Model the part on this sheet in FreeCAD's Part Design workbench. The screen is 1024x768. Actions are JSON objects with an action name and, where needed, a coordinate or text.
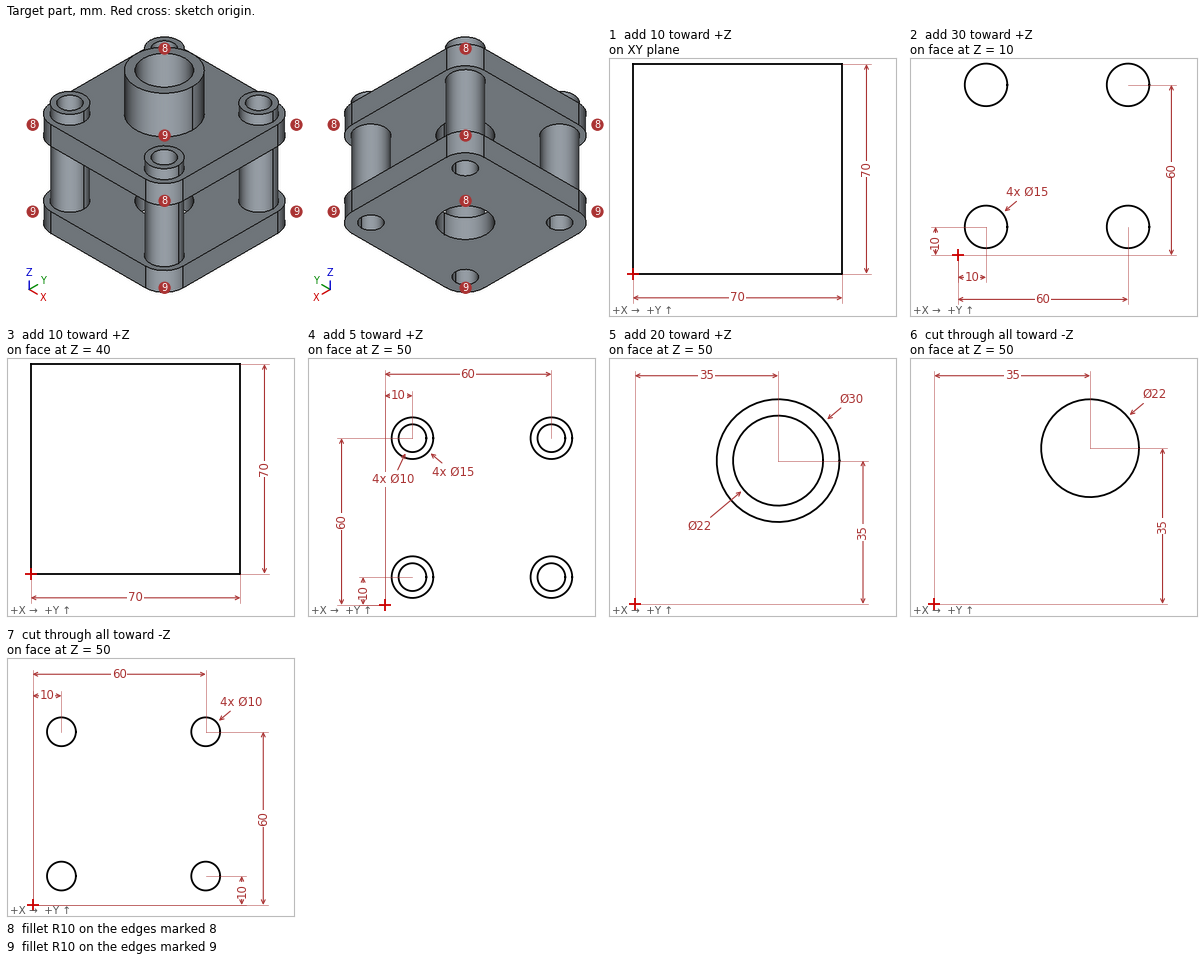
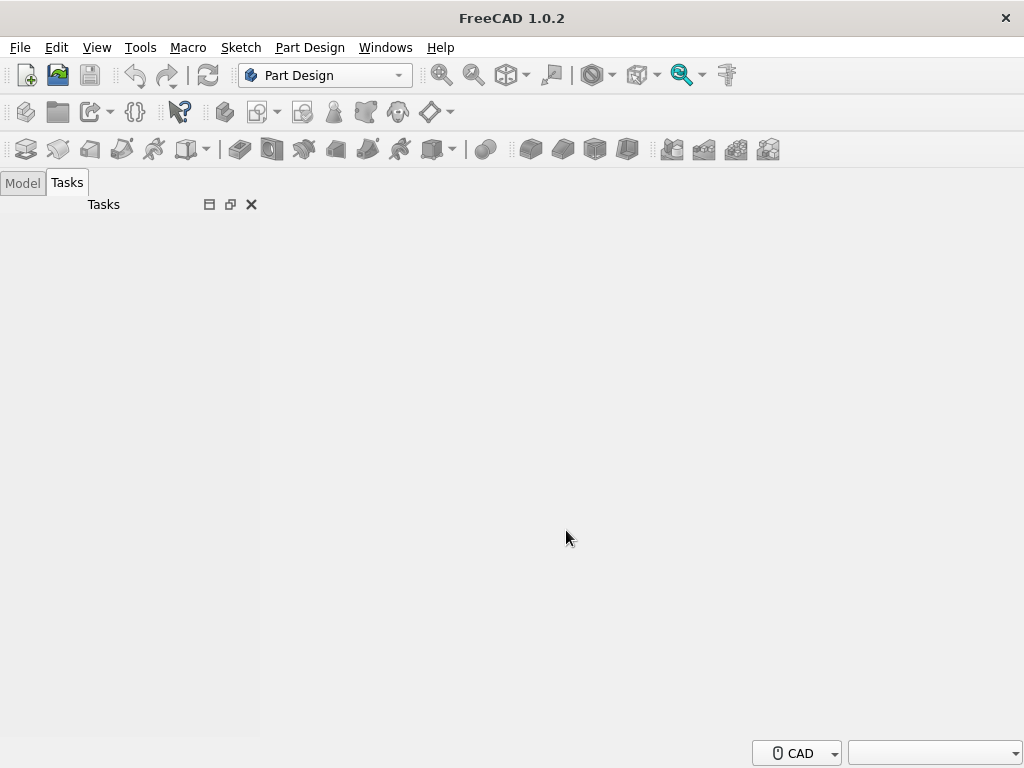
{"action": "key", "text": "ctrl+n"}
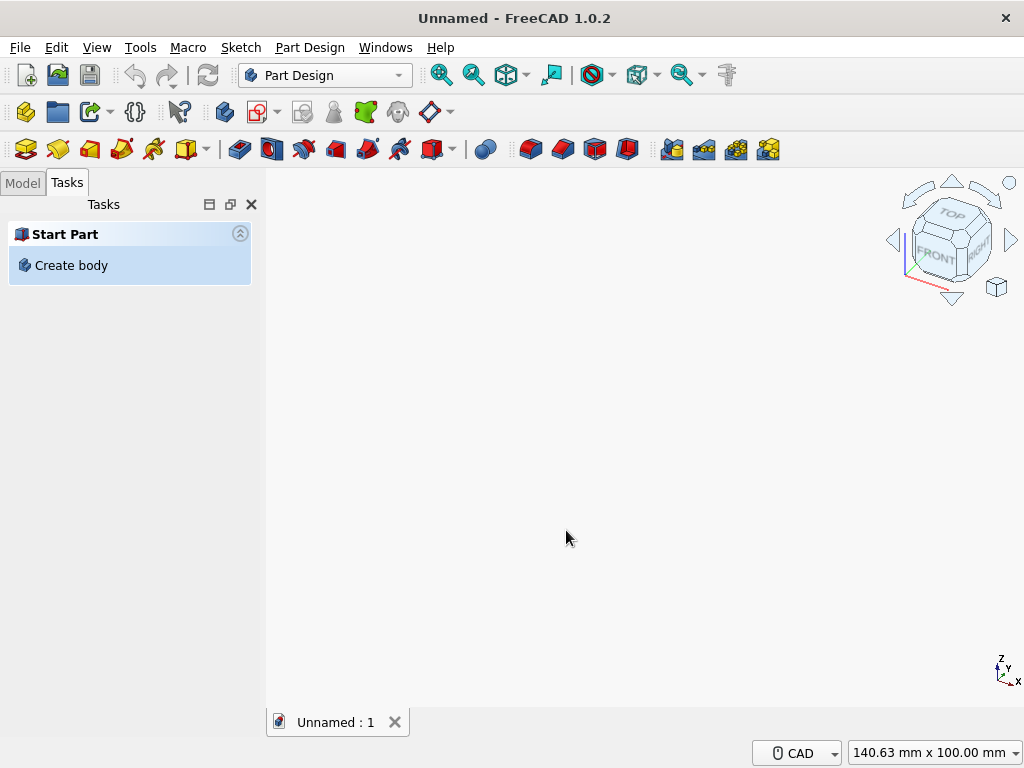
{"action": "left_click", "coordinate": [258, 112]}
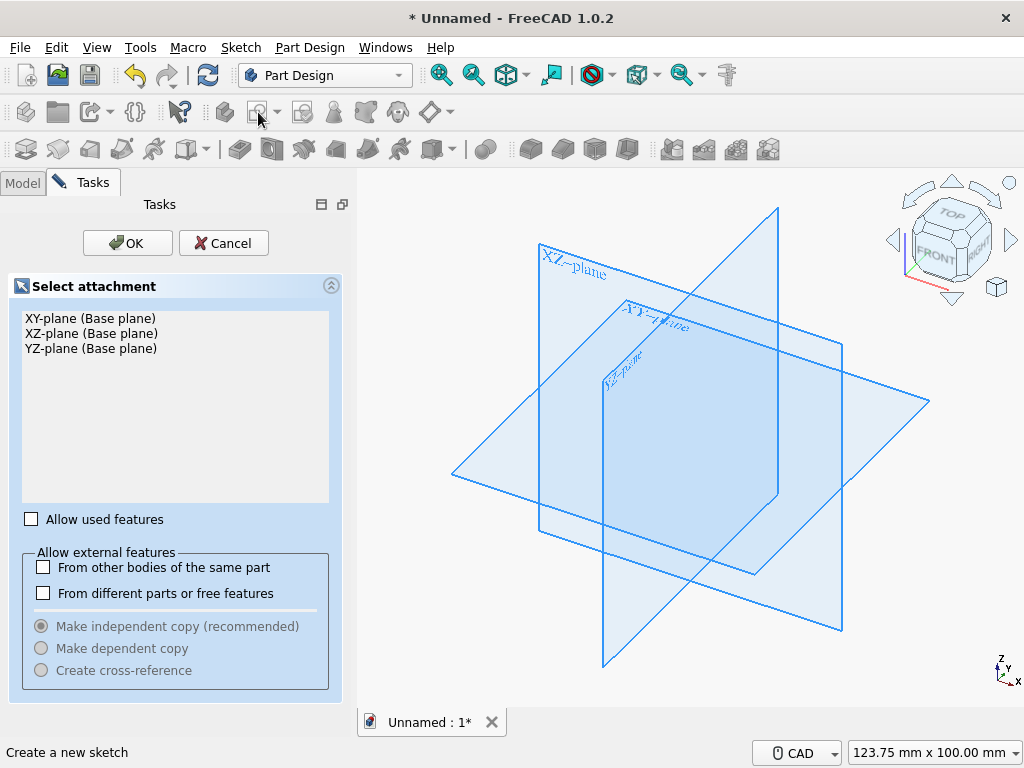
{"action": "left_click", "coordinate": [82, 318]}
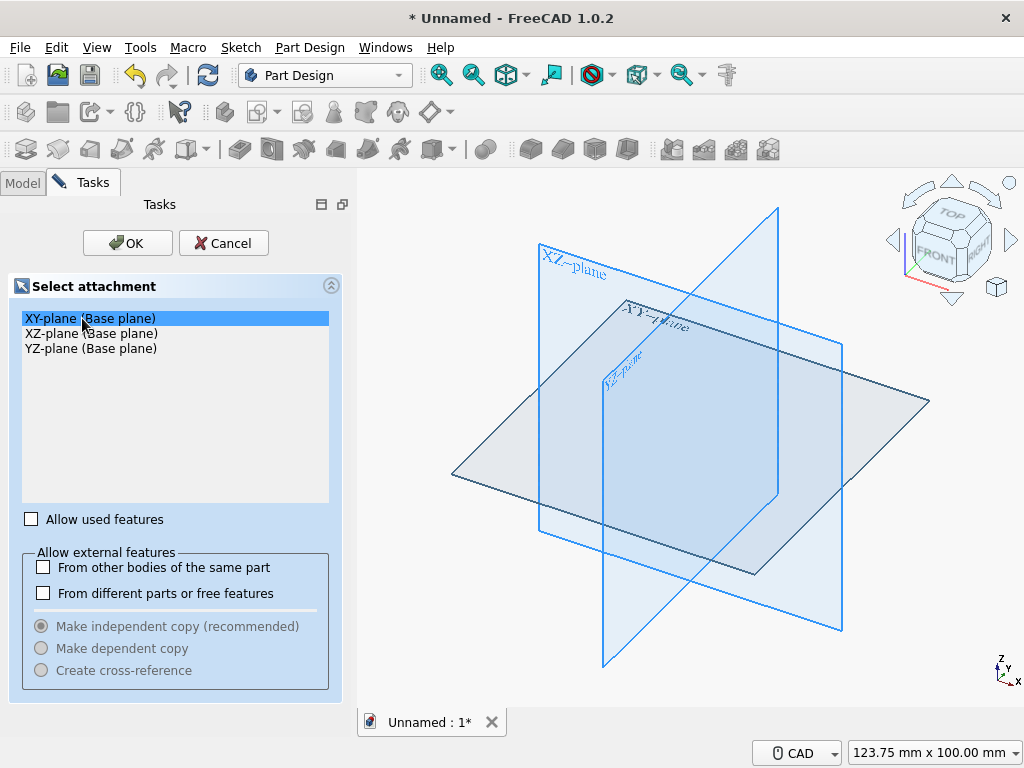
{"action": "left_click", "coordinate": [128, 243]}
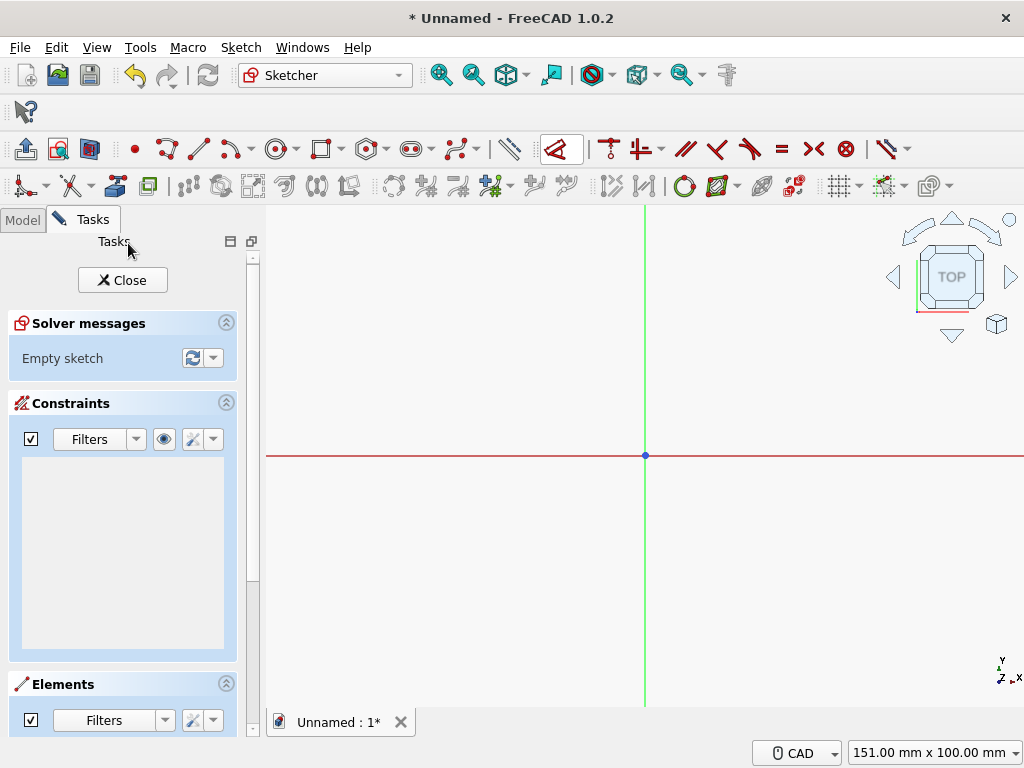
{"action": "scroll", "coordinate": [294, 679], "scroll_direction": "down", "scroll_amount": 2}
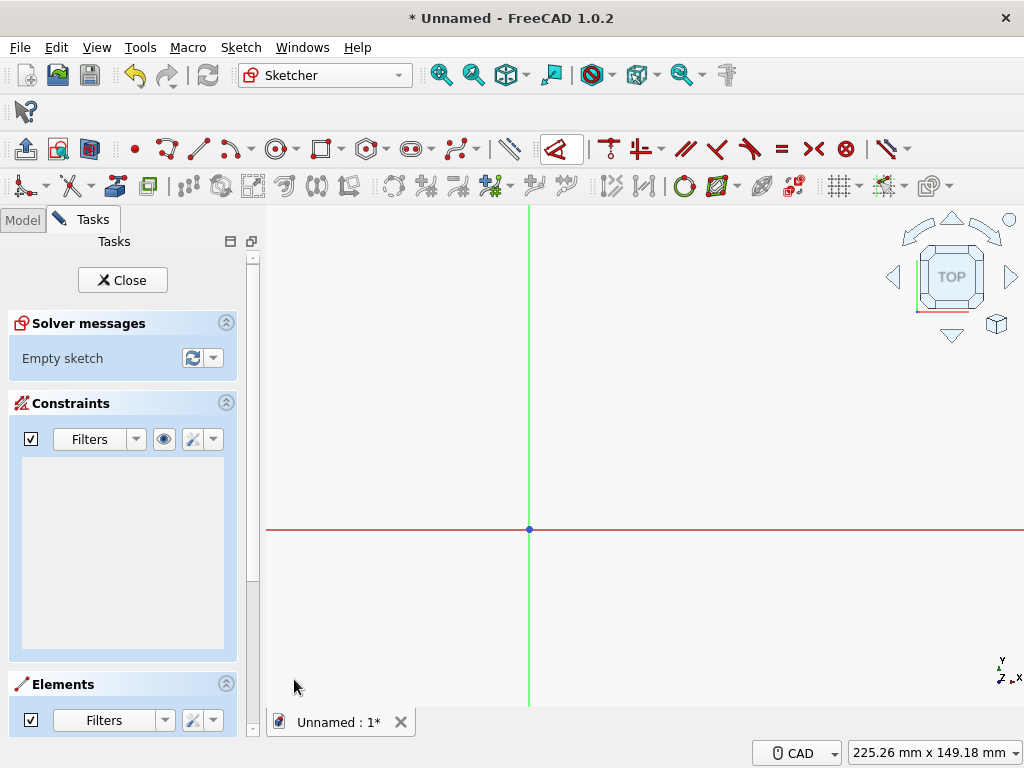
{"action": "key", "text": "g r"}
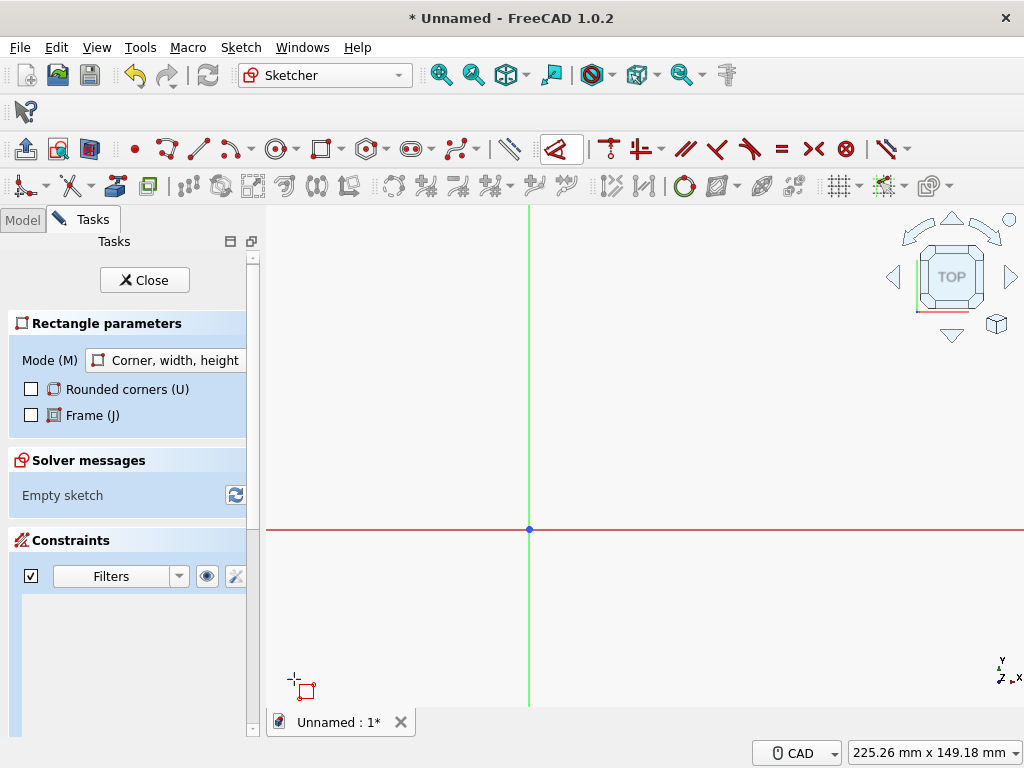
{"action": "left_click", "coordinate": [529, 530]}
{"action": "left_click", "coordinate": [765, 294]}
{"action": "key", "text": "Escape"}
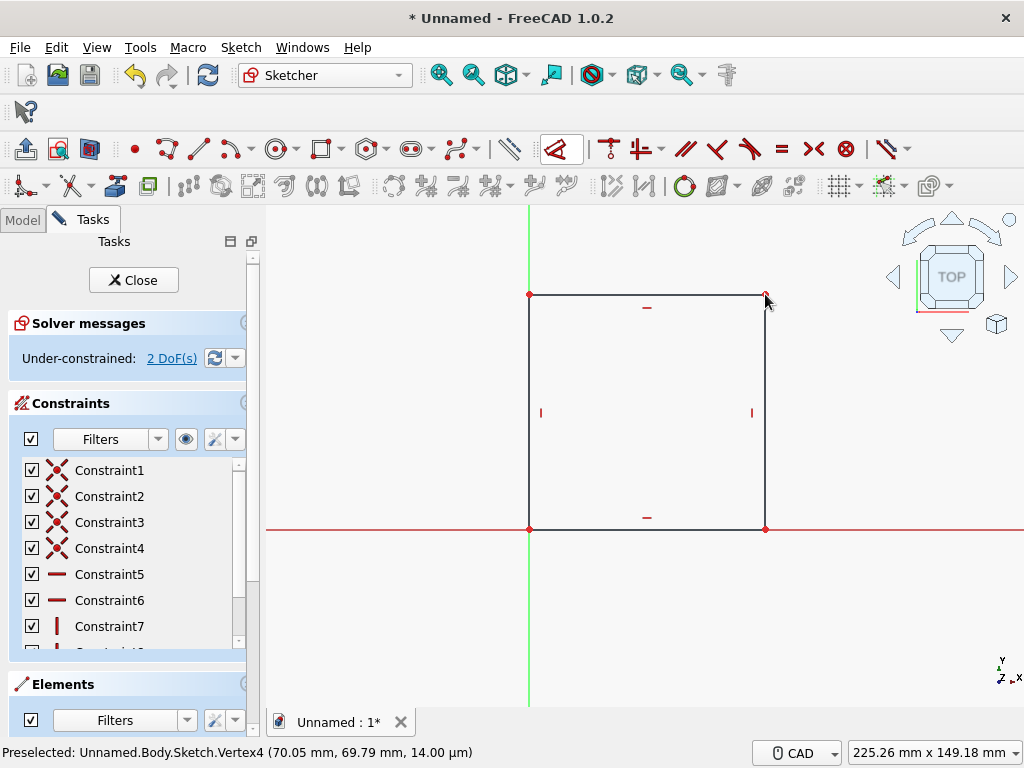
{"action": "left_click", "coordinate": [556, 150]}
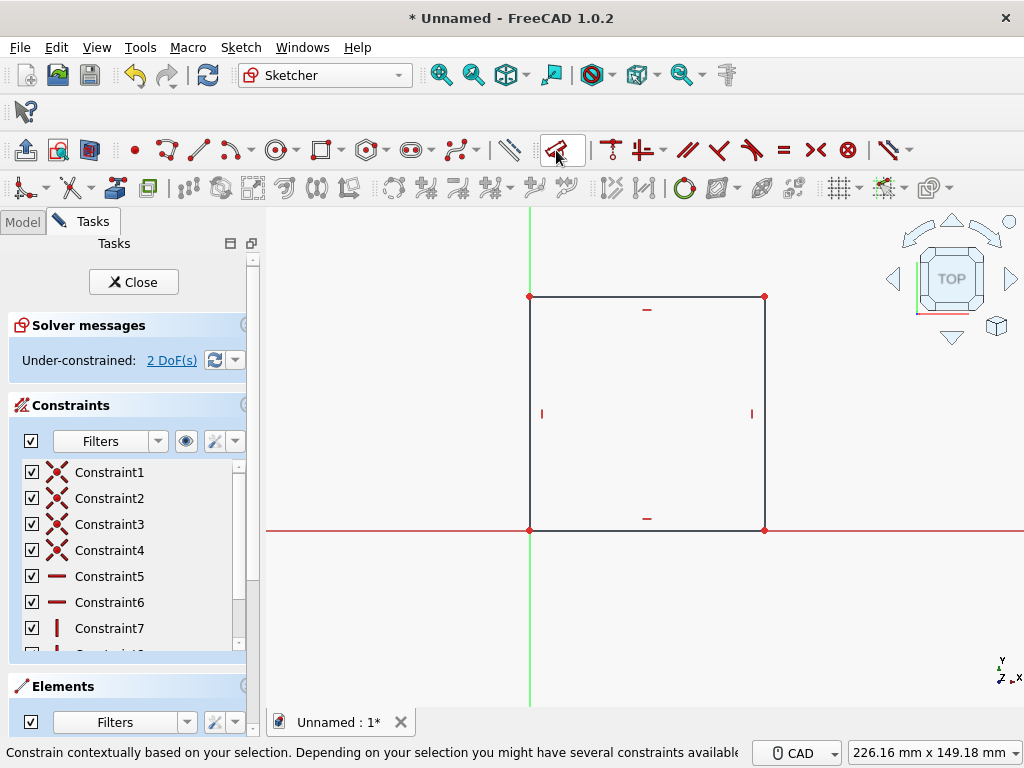
{"action": "left_click", "coordinate": [600, 531]}
{"action": "left_click", "coordinate": [647, 565]}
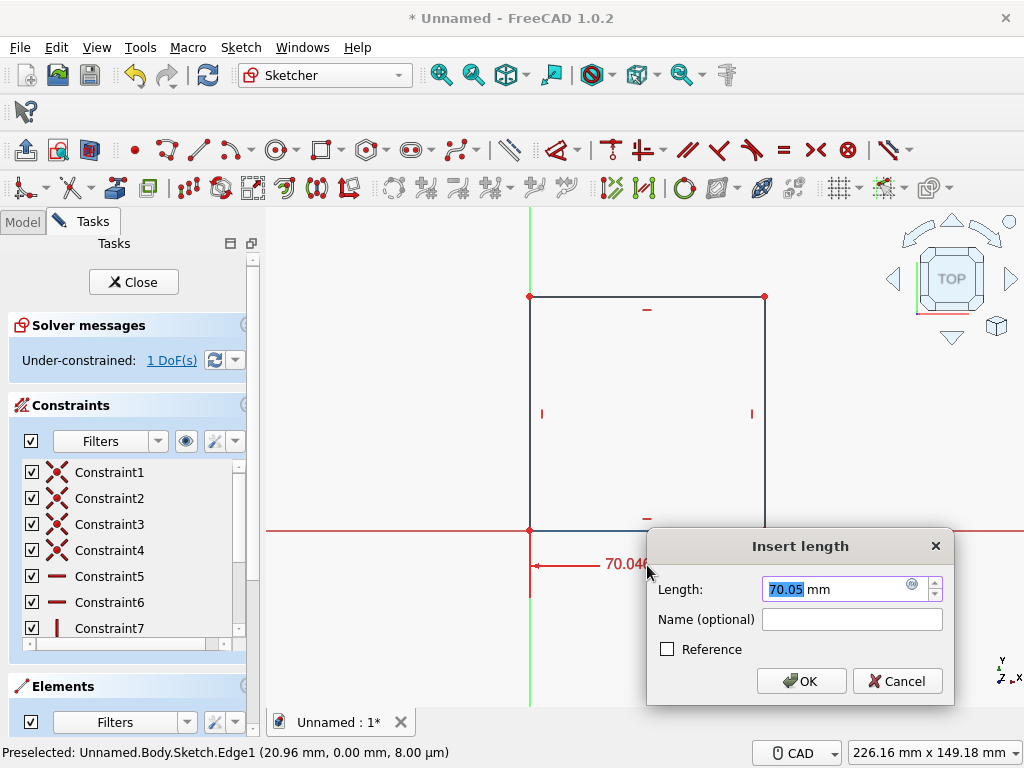
{"action": "type", "text": "70"}
{"action": "key", "text": "Return"}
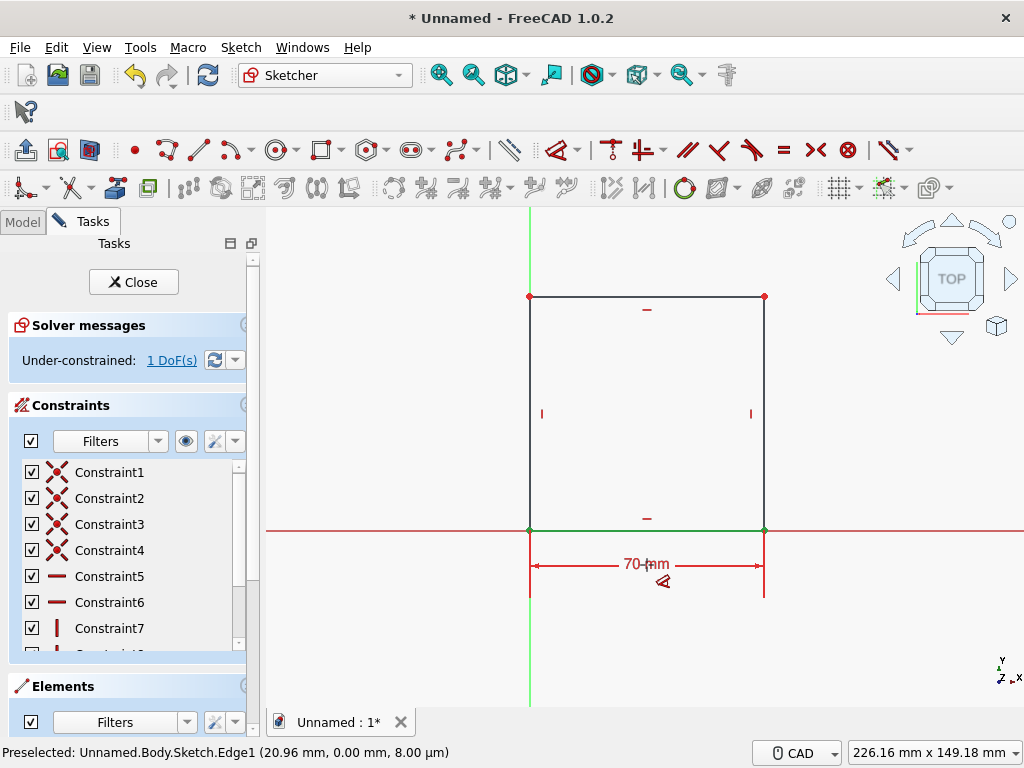
{"action": "left_click", "coordinate": [764, 460]}
{"action": "left_click", "coordinate": [798, 414]}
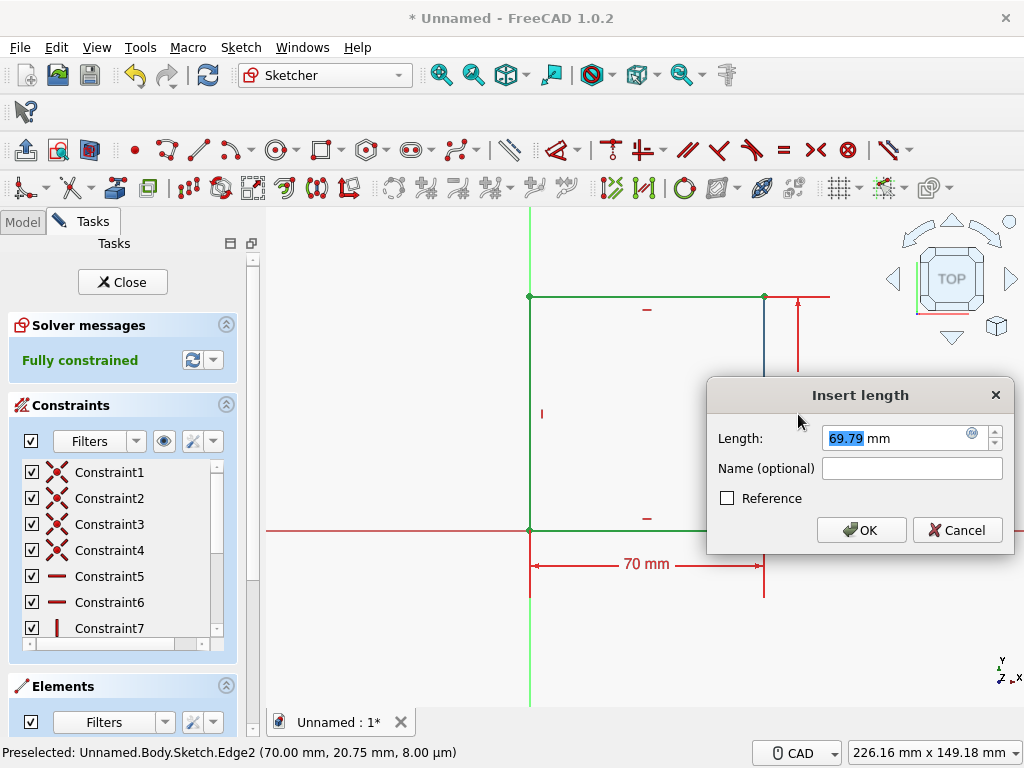
{"action": "type", "text": "70"}
{"action": "key", "text": "Return"}
{"action": "key", "text": "Escape"}